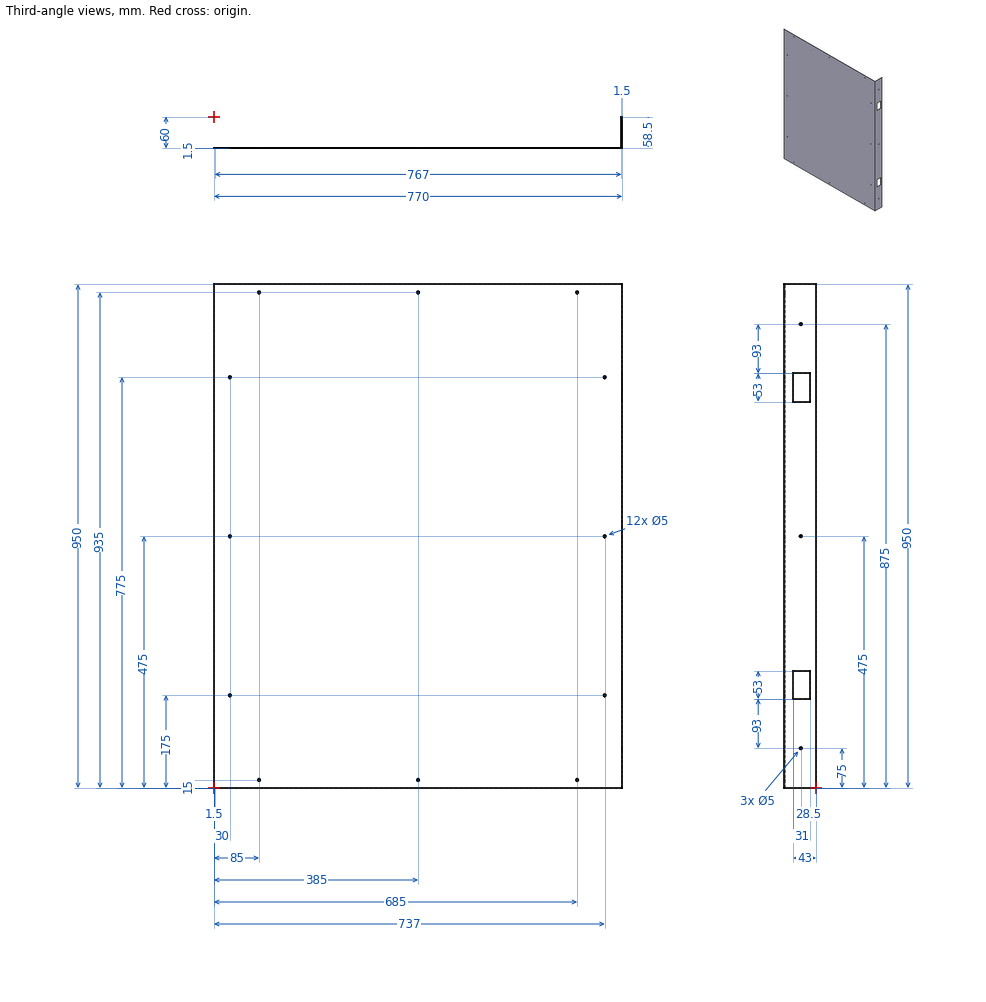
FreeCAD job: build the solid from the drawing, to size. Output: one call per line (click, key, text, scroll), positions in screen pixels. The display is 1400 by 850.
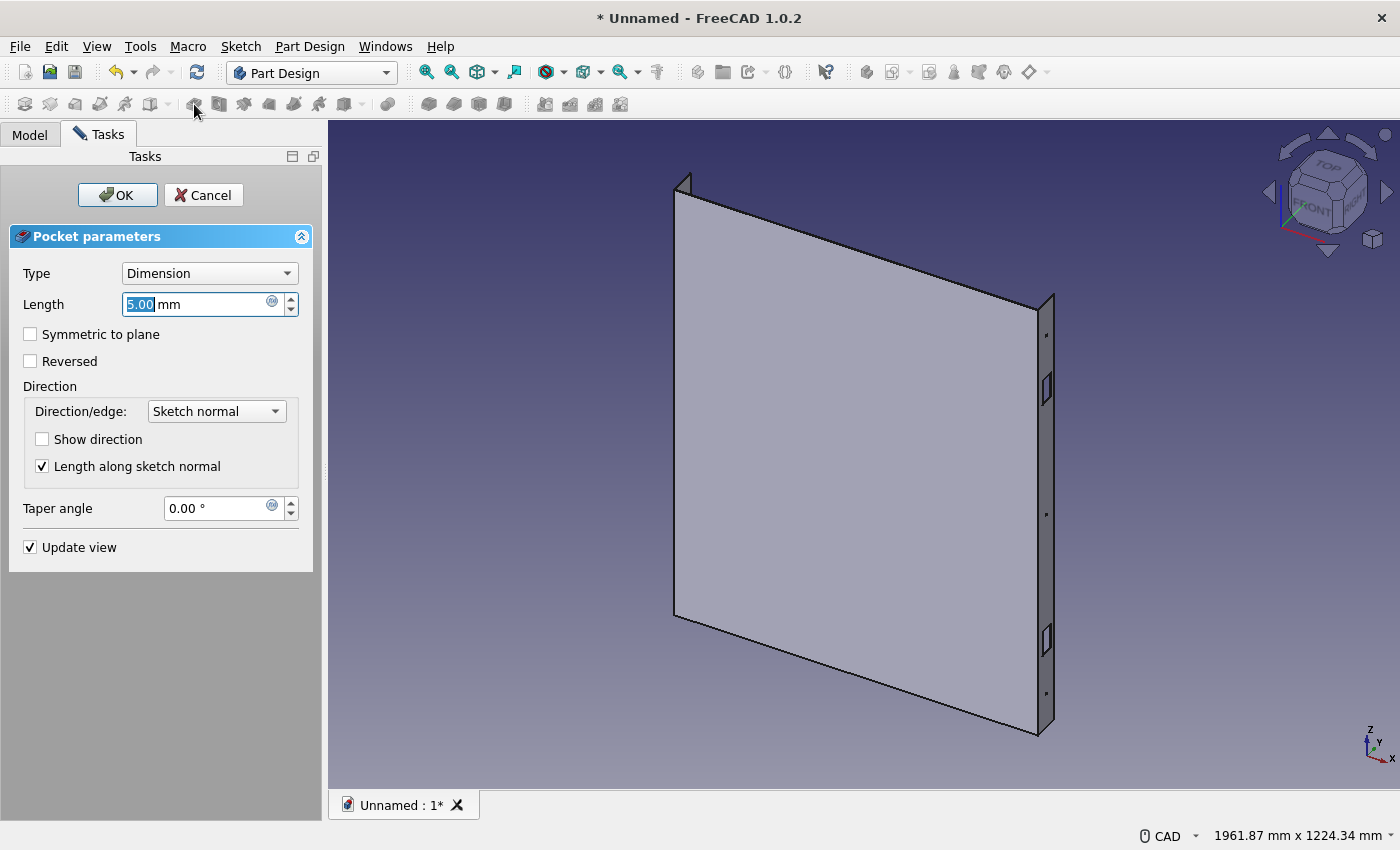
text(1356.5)
key(Tab)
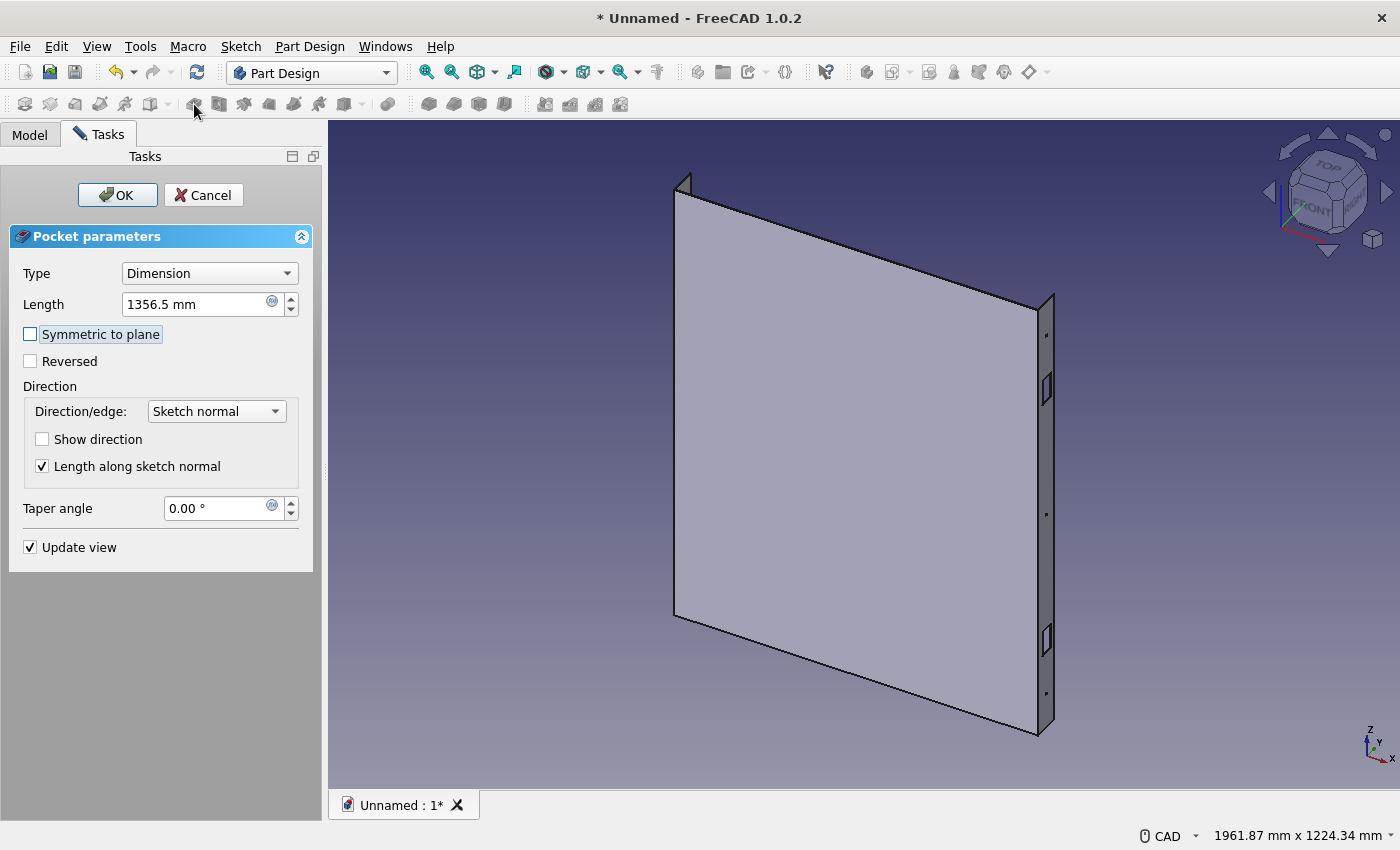
click(118, 195)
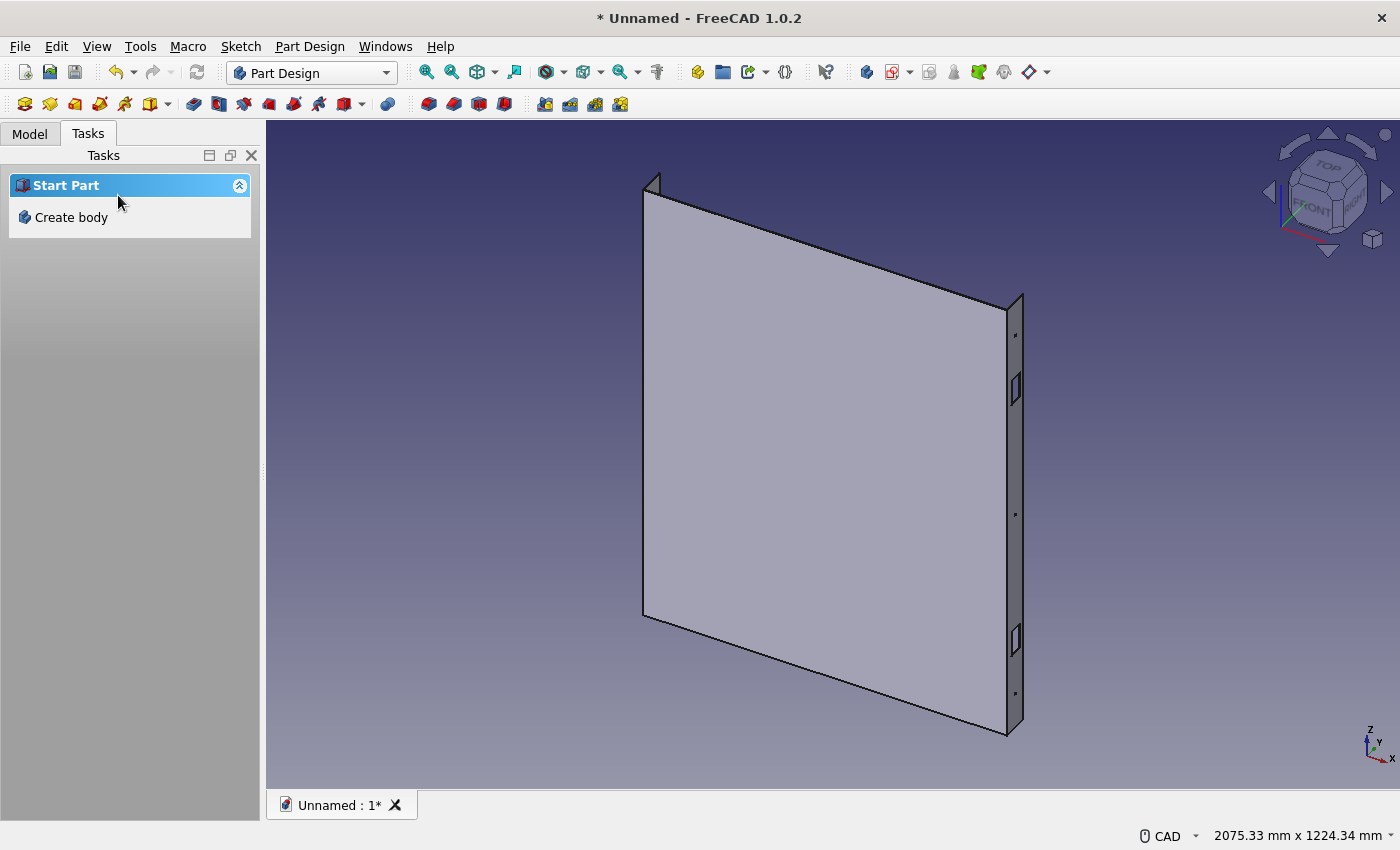
click(825, 462)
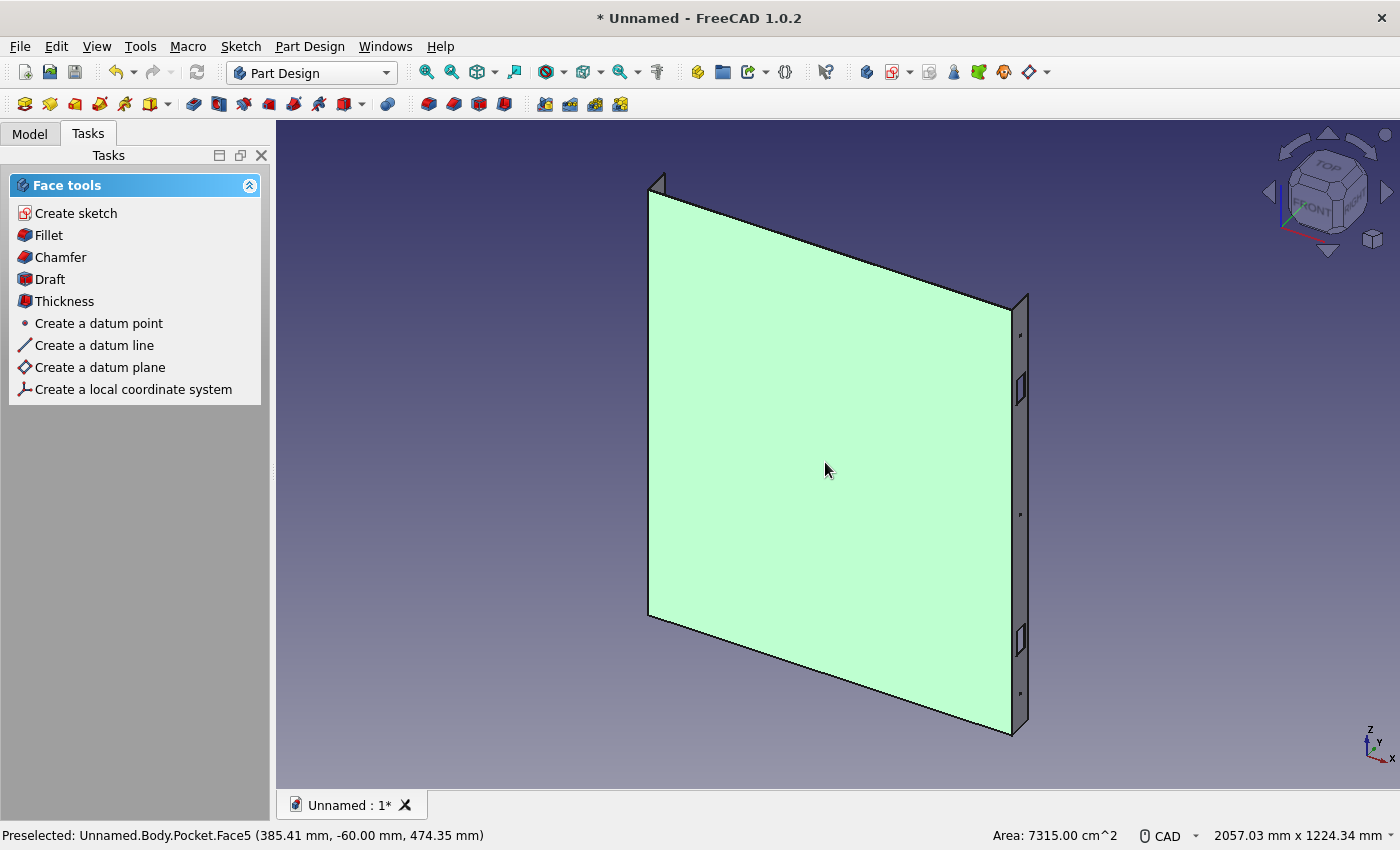
click(892, 72)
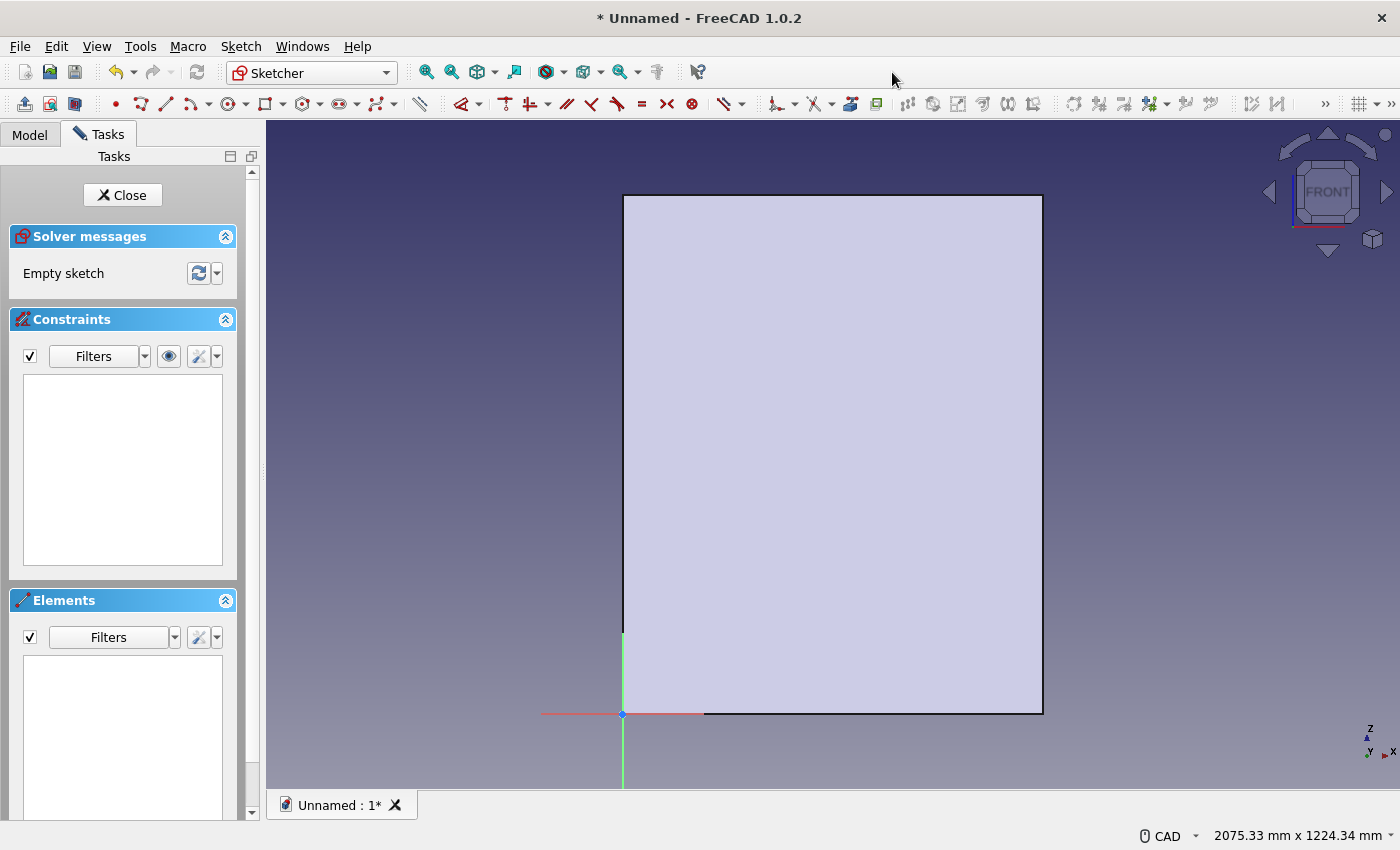
click(228, 104)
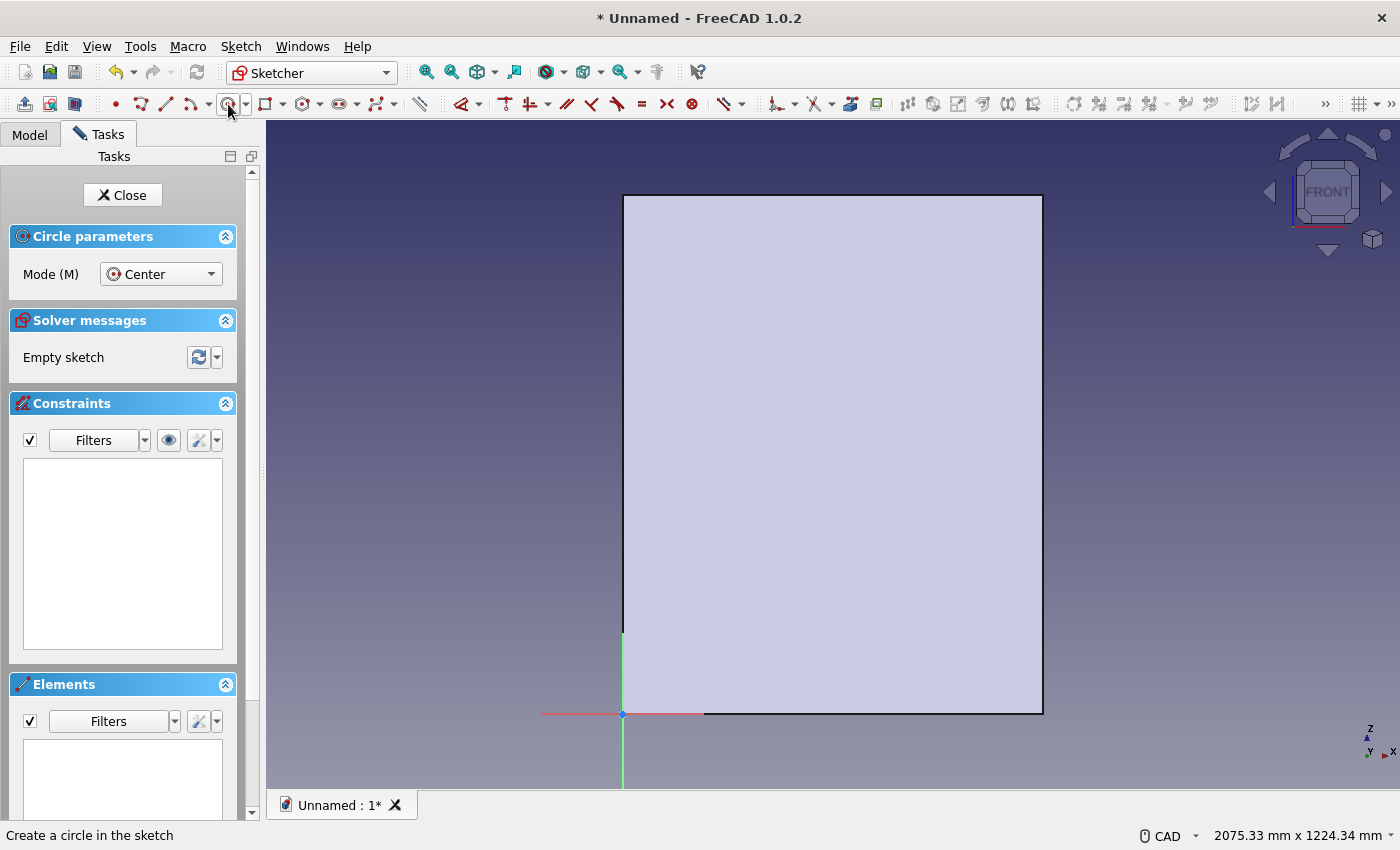
scroll(1025, 455, up, 15)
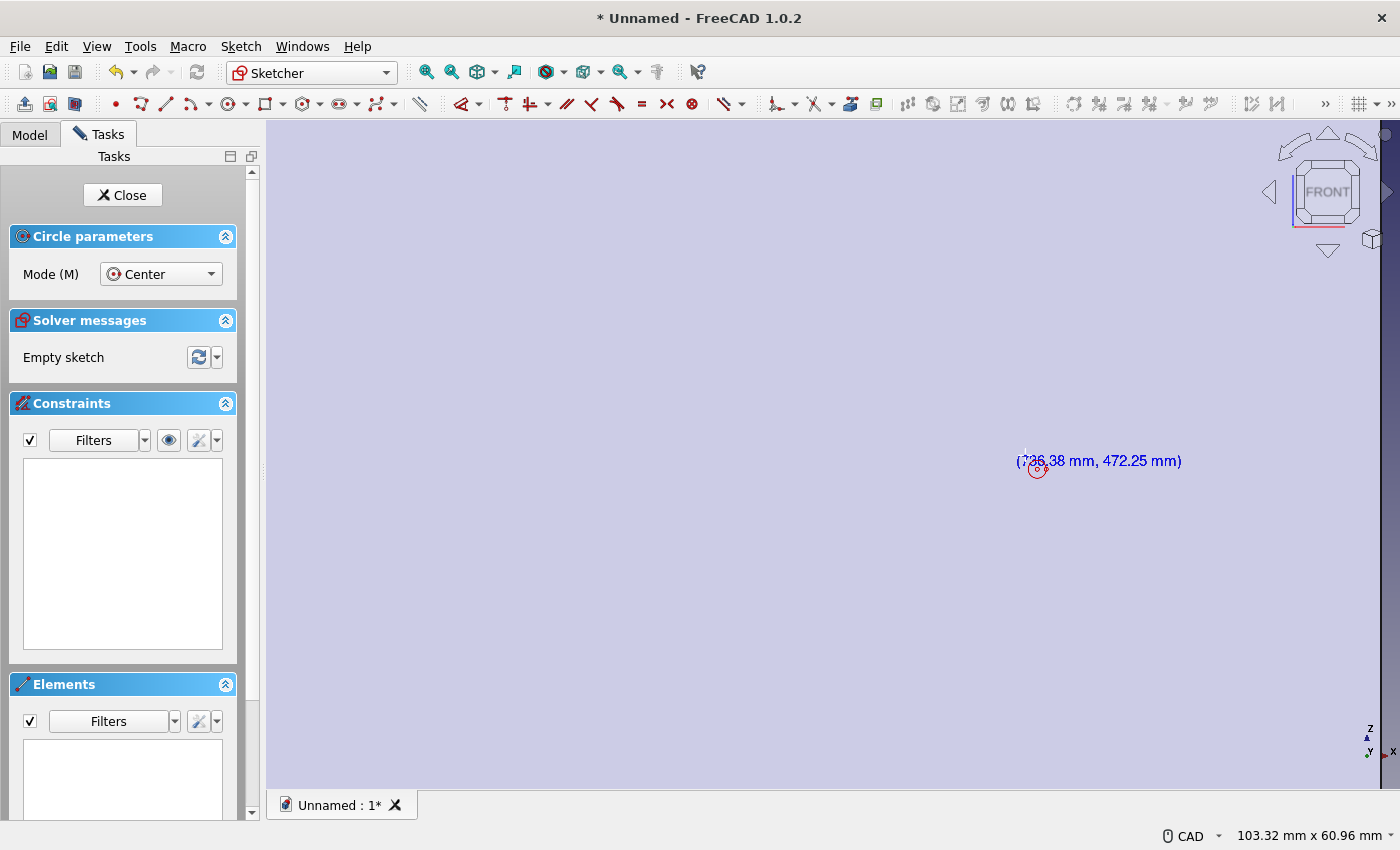
scroll(962, 452, down, 15)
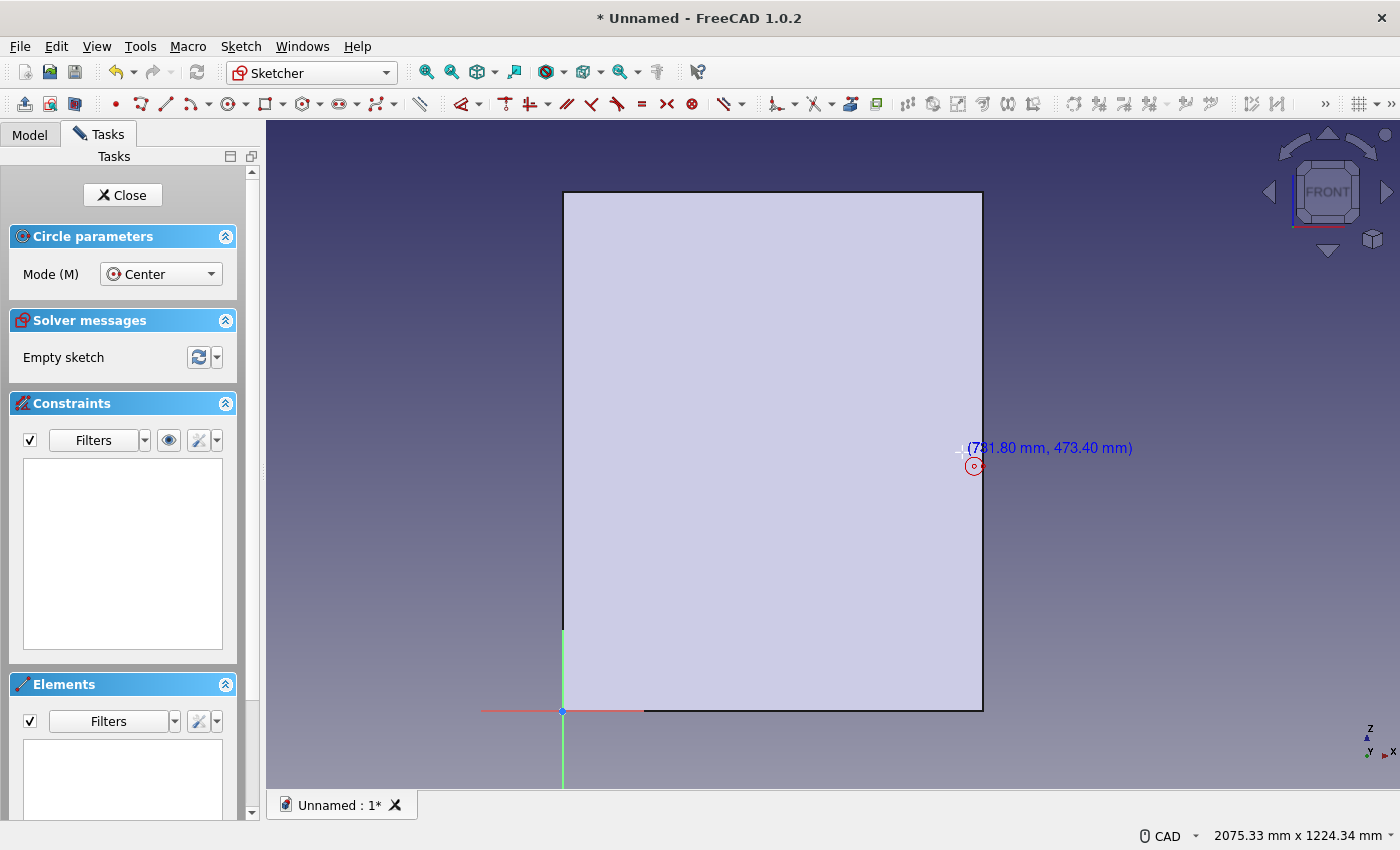
click(965, 452)